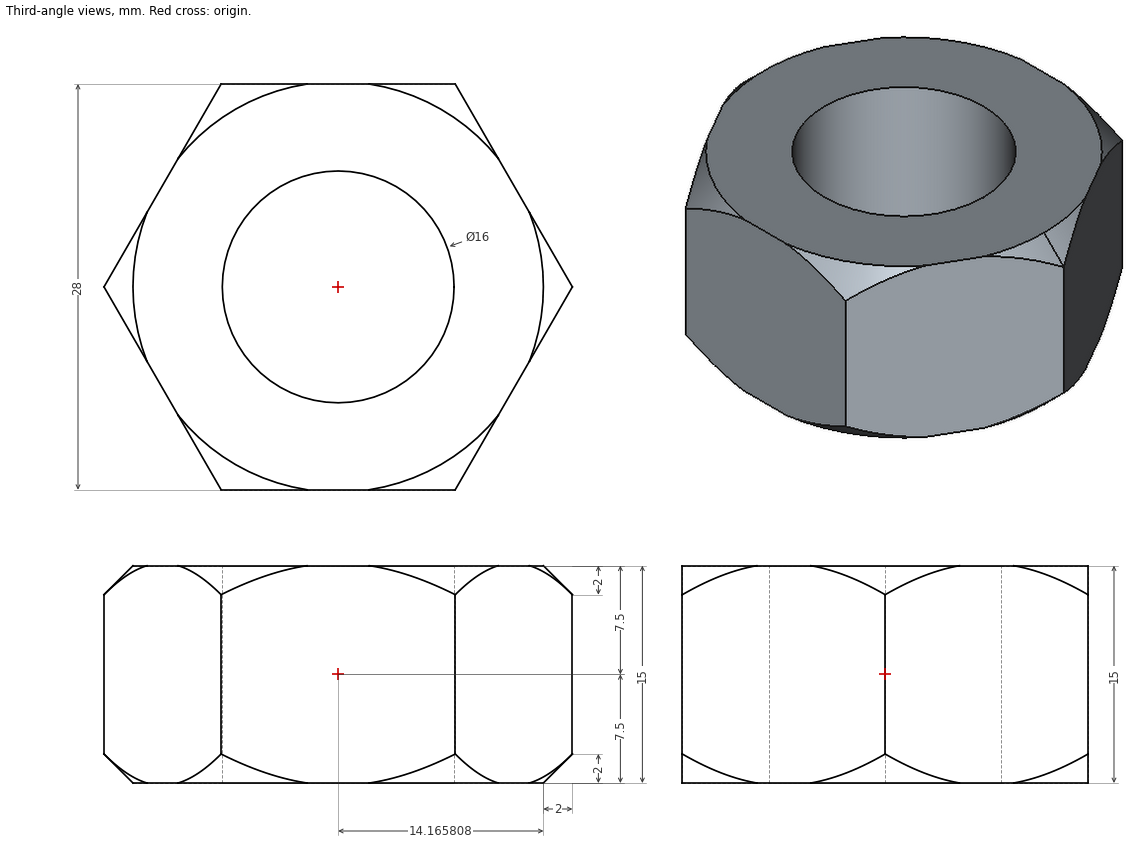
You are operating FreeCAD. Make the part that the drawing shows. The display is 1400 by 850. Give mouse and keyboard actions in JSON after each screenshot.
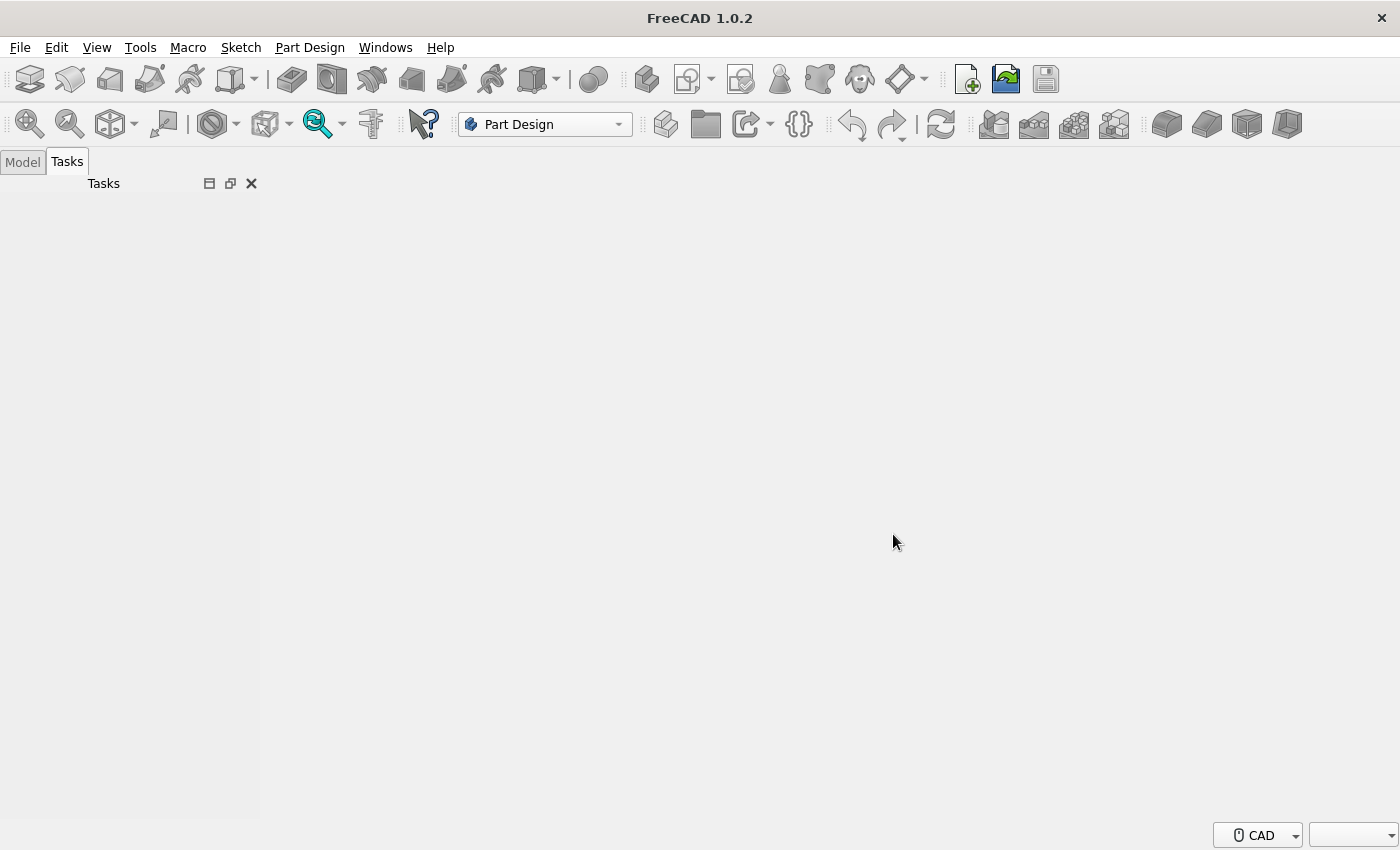
{"action": "left_click", "coordinate": [966, 80]}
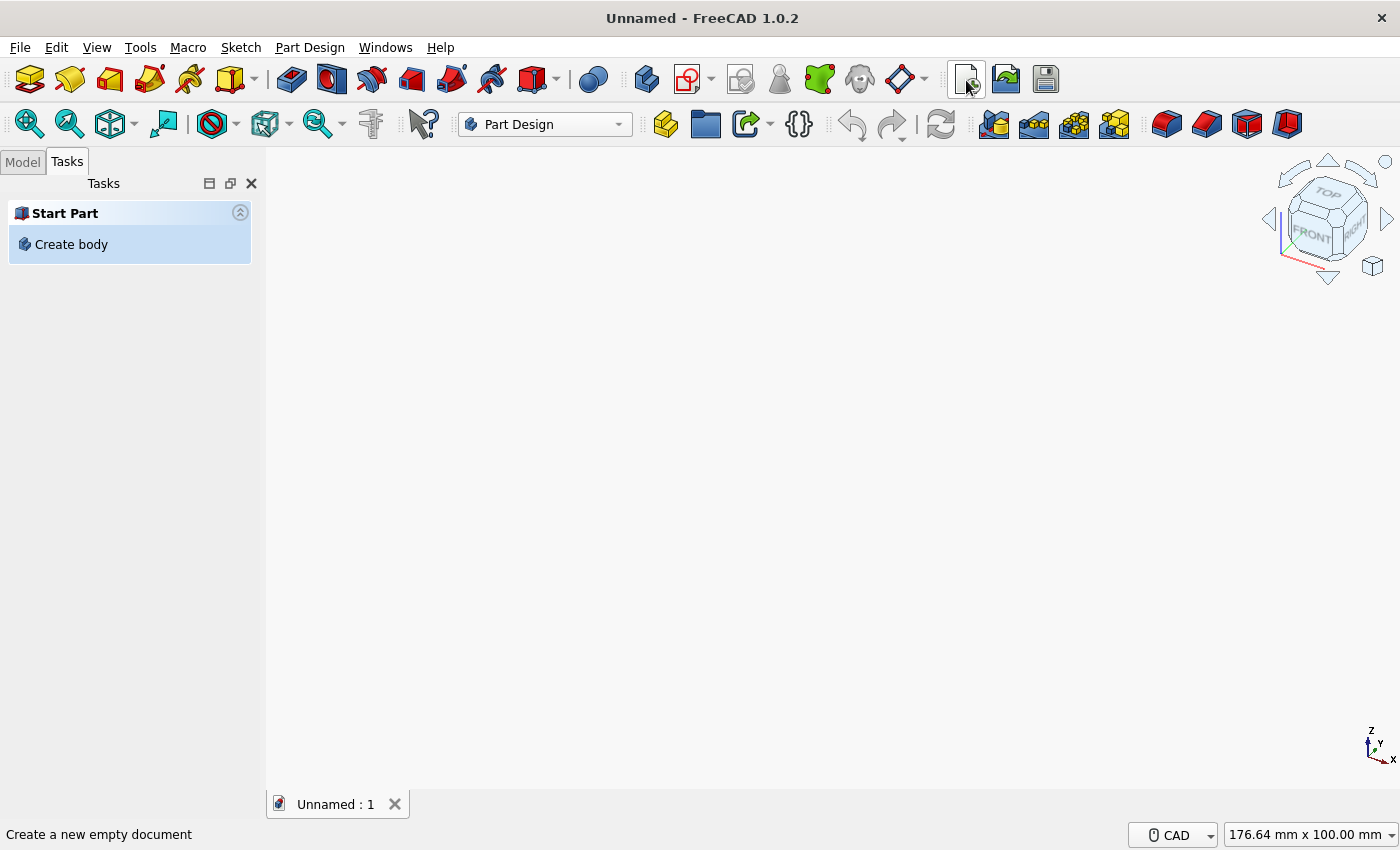
{"action": "left_click", "coordinate": [688, 80]}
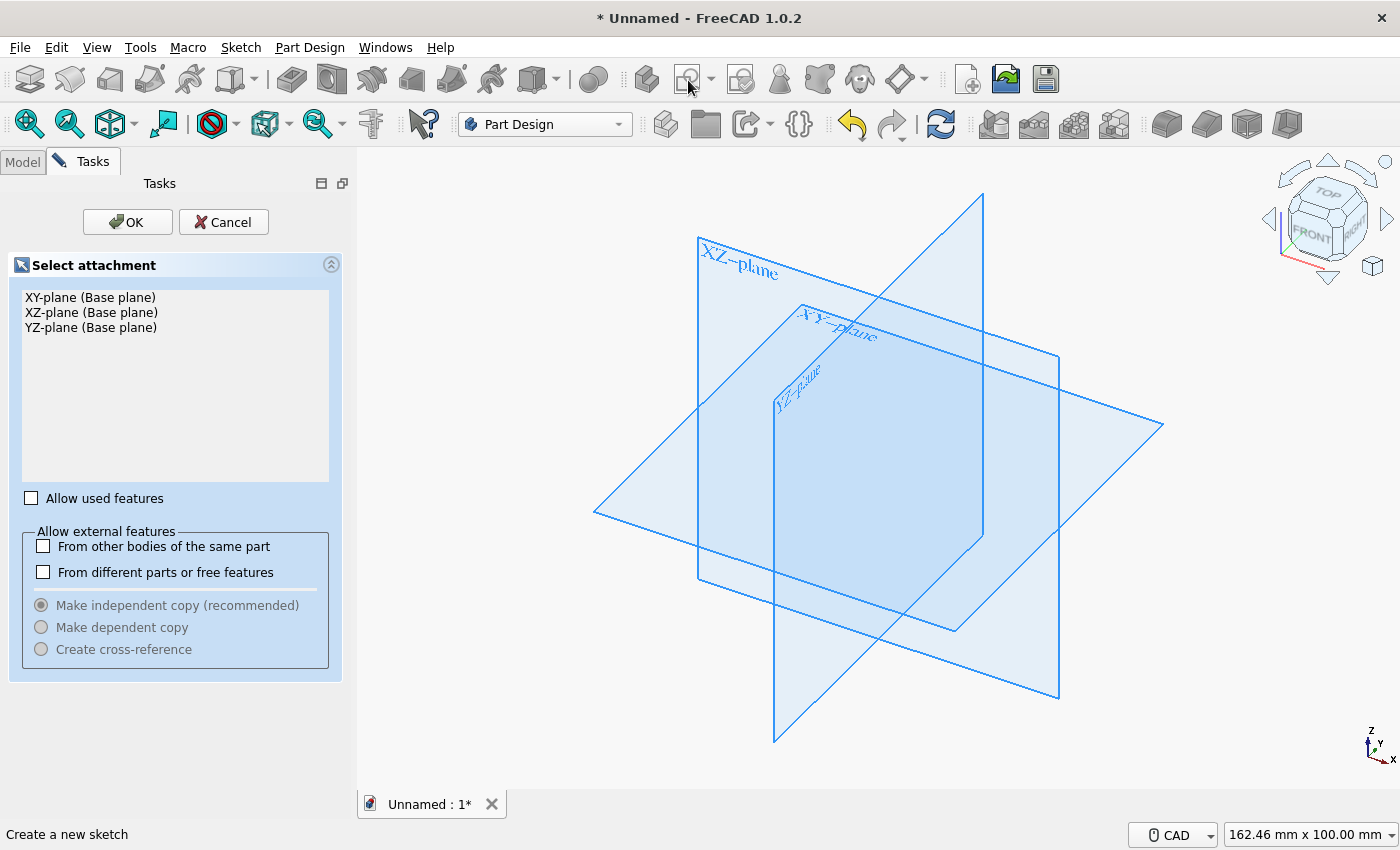
{"action": "left_click", "coordinate": [82, 298]}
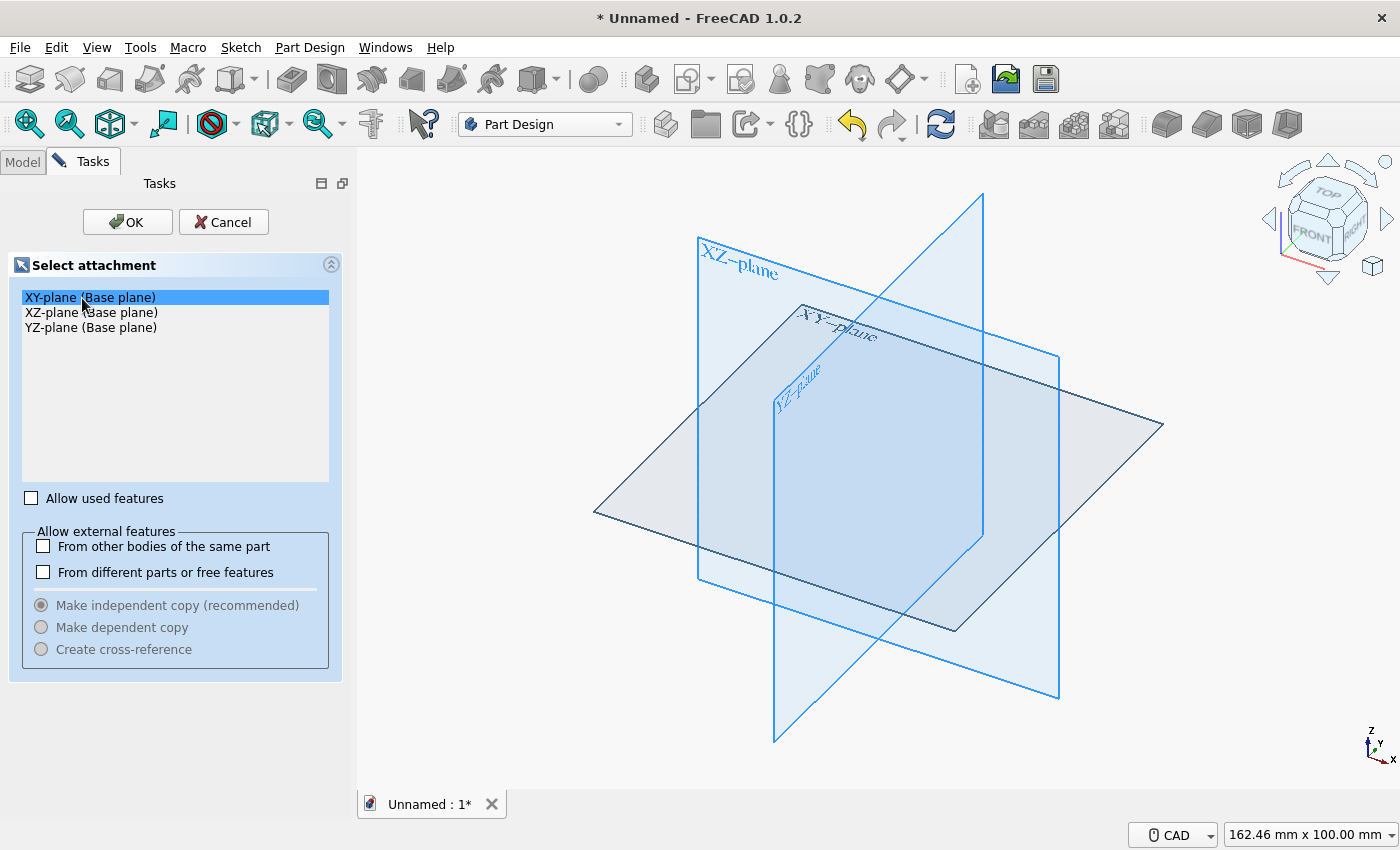
{"action": "left_click", "coordinate": [128, 222]}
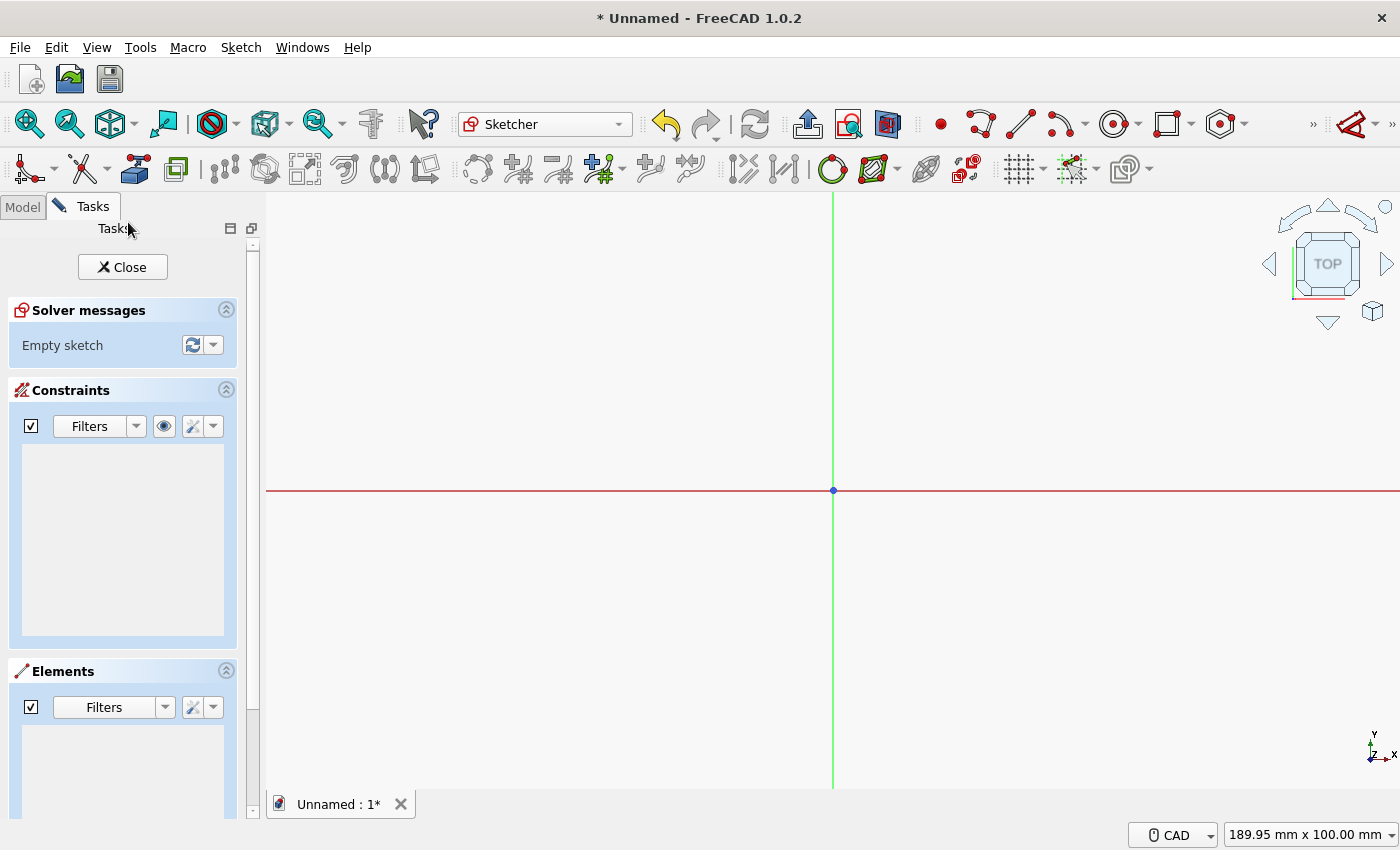
{"action": "scroll", "coordinate": [889, 491], "scroll_direction": "up", "scroll_amount": 4}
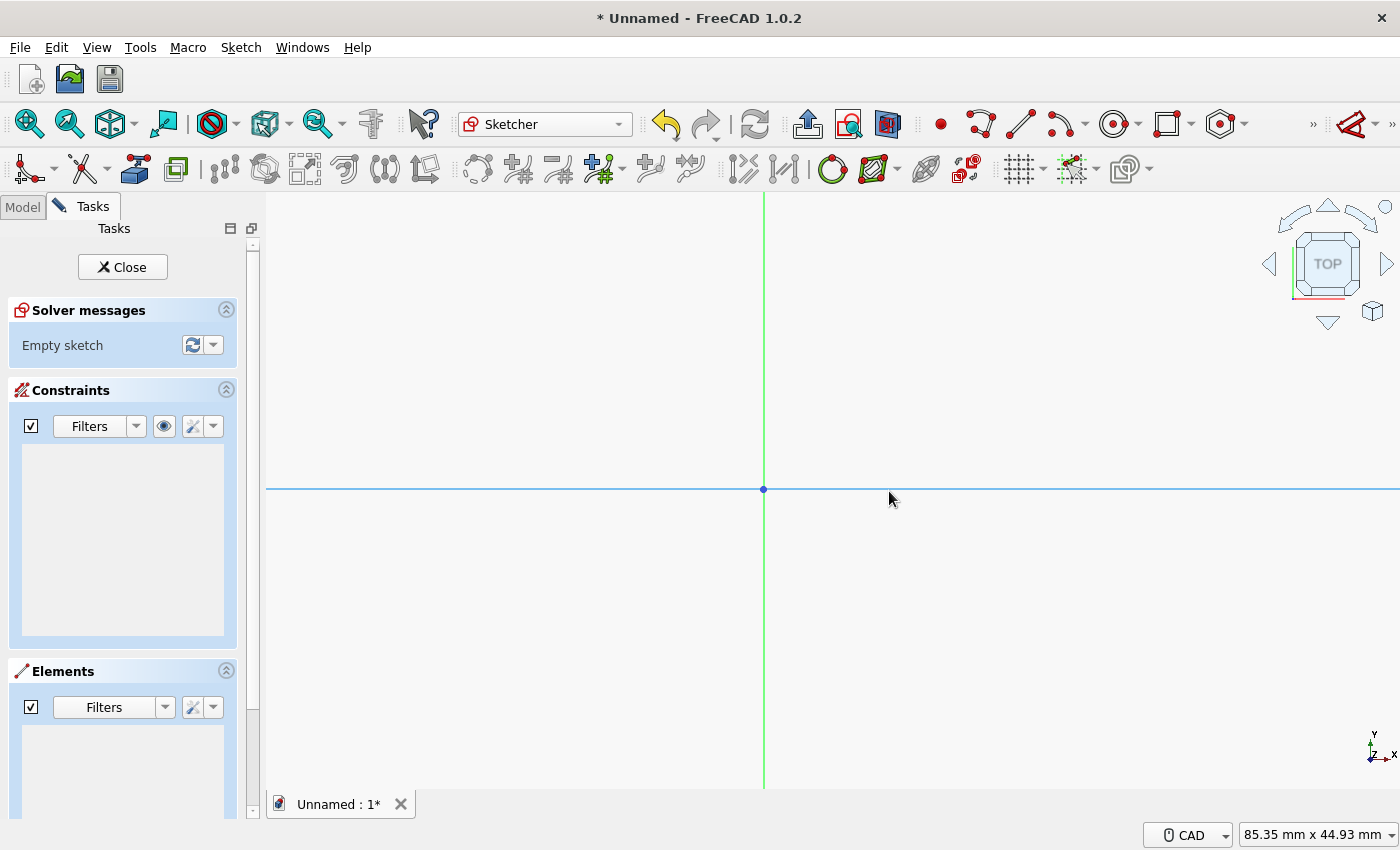
{"action": "left_click", "coordinate": [1220, 124]}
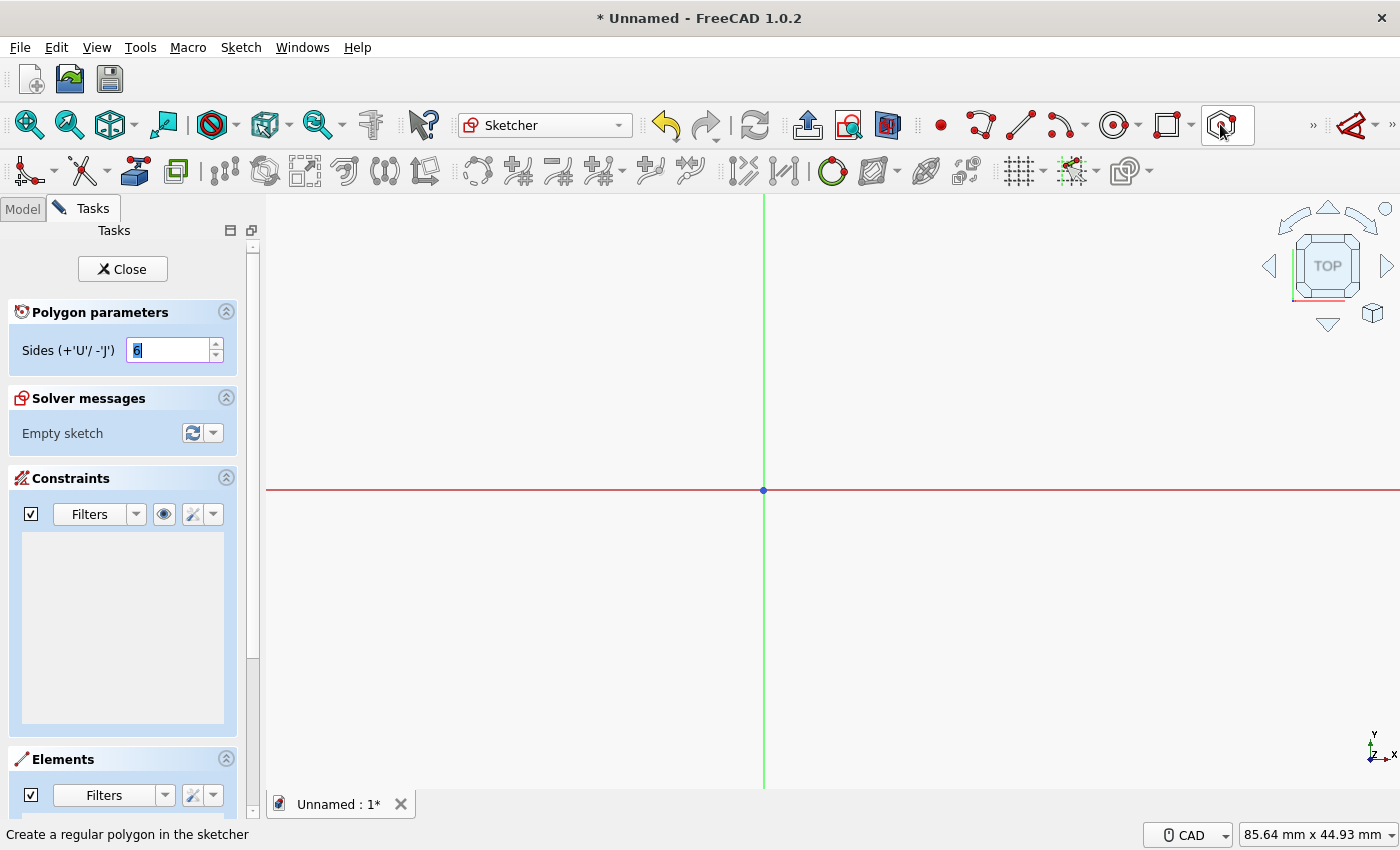
{"action": "left_click", "coordinate": [764, 490]}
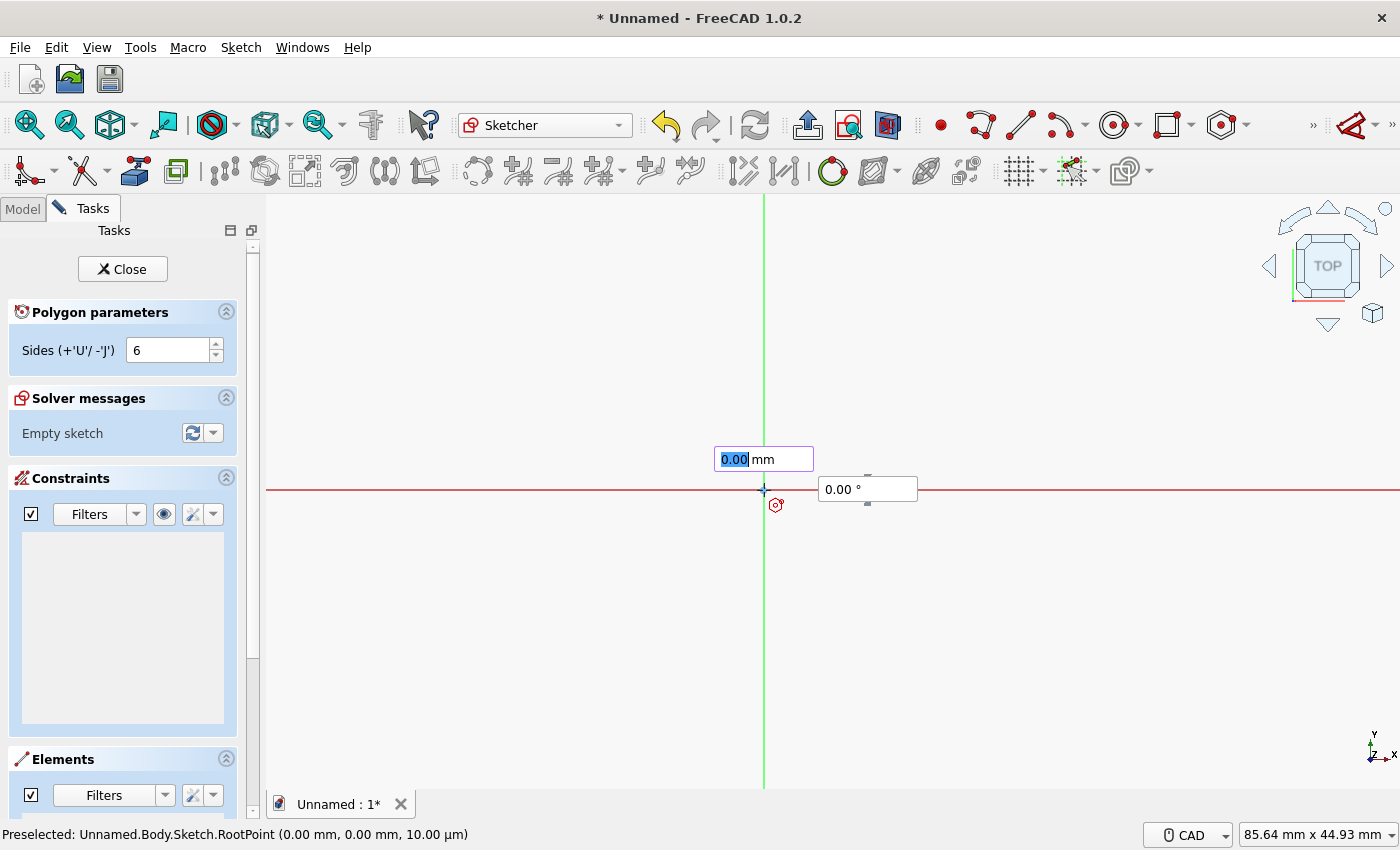
{"action": "left_click", "coordinate": [978, 490]}
{"action": "right_click", "coordinate": [978, 490]}